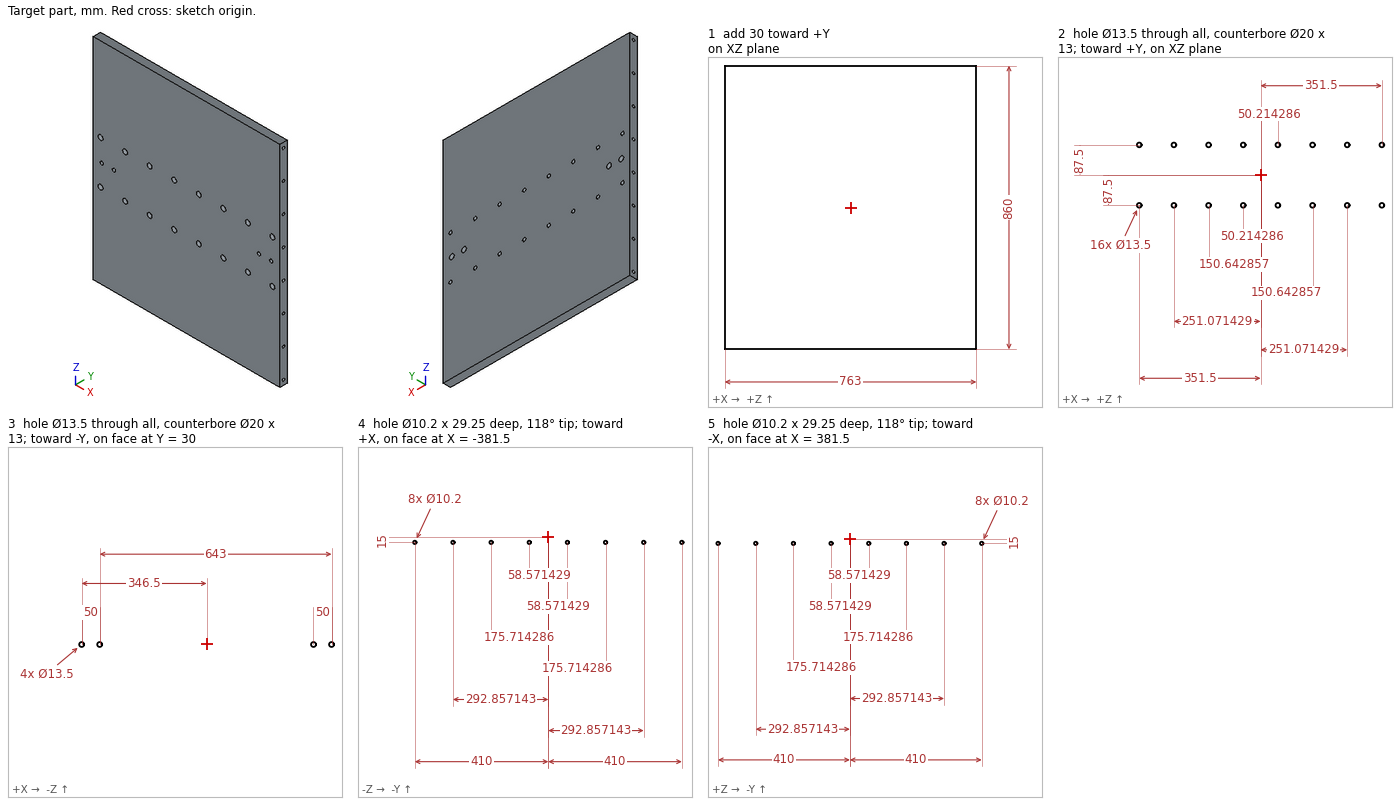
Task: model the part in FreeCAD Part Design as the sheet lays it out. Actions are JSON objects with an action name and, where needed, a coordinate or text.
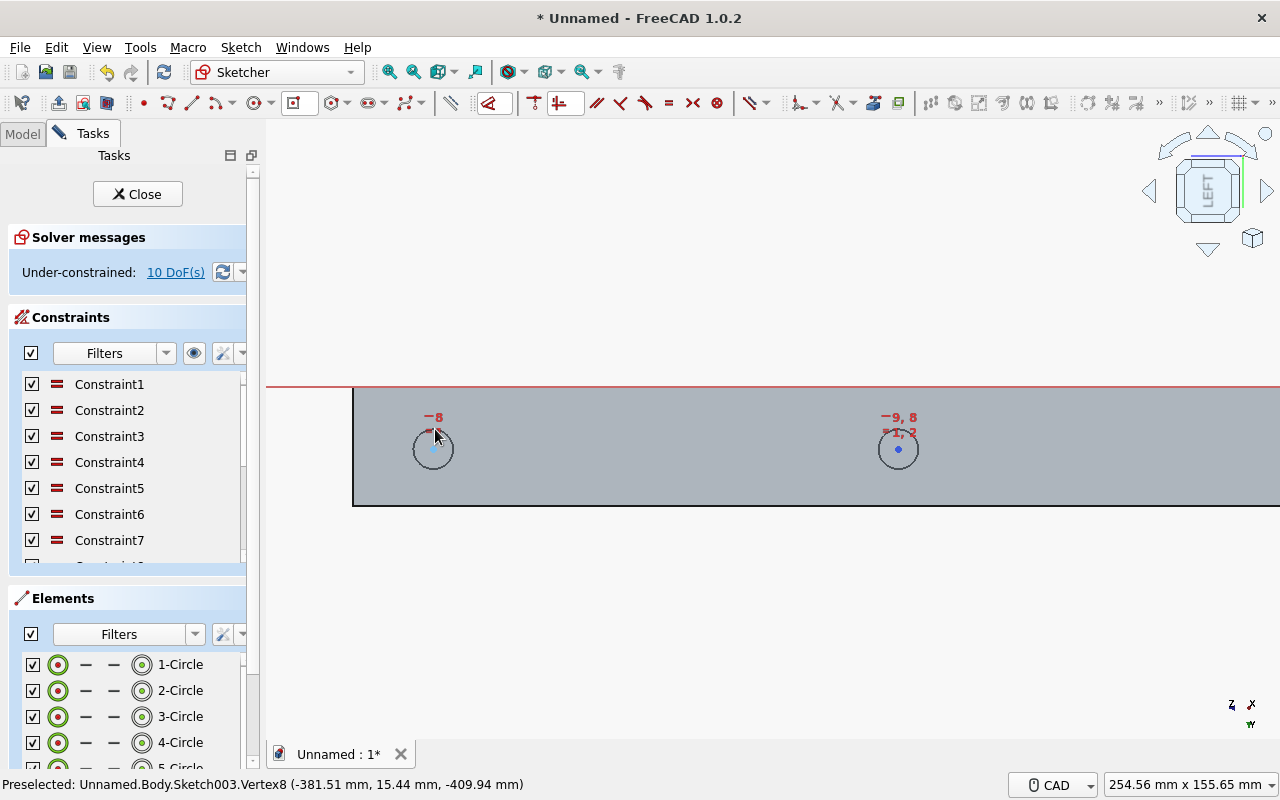
{"action": "left_click", "coordinate": [433, 469]}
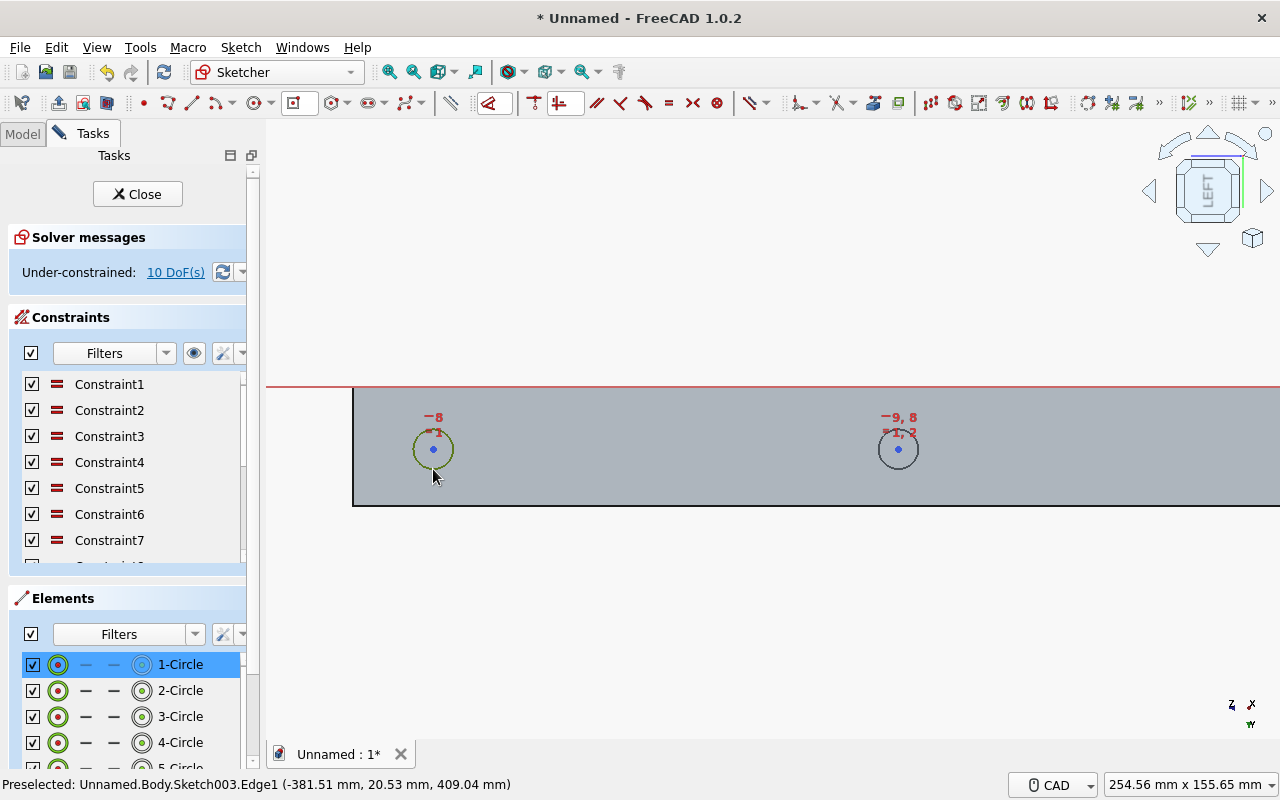
{"action": "key", "text": "k o"}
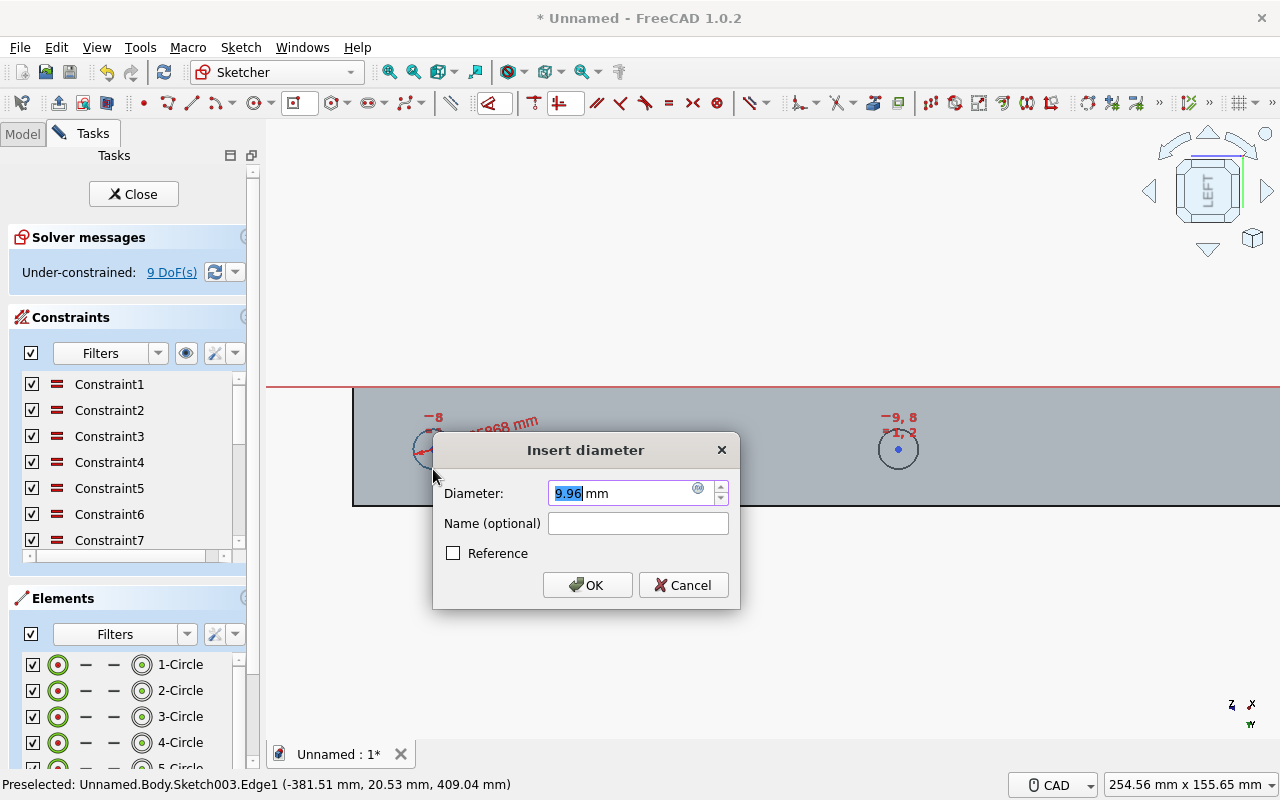
{"action": "type", "text": "10.2"}
{"action": "key", "text": "Return"}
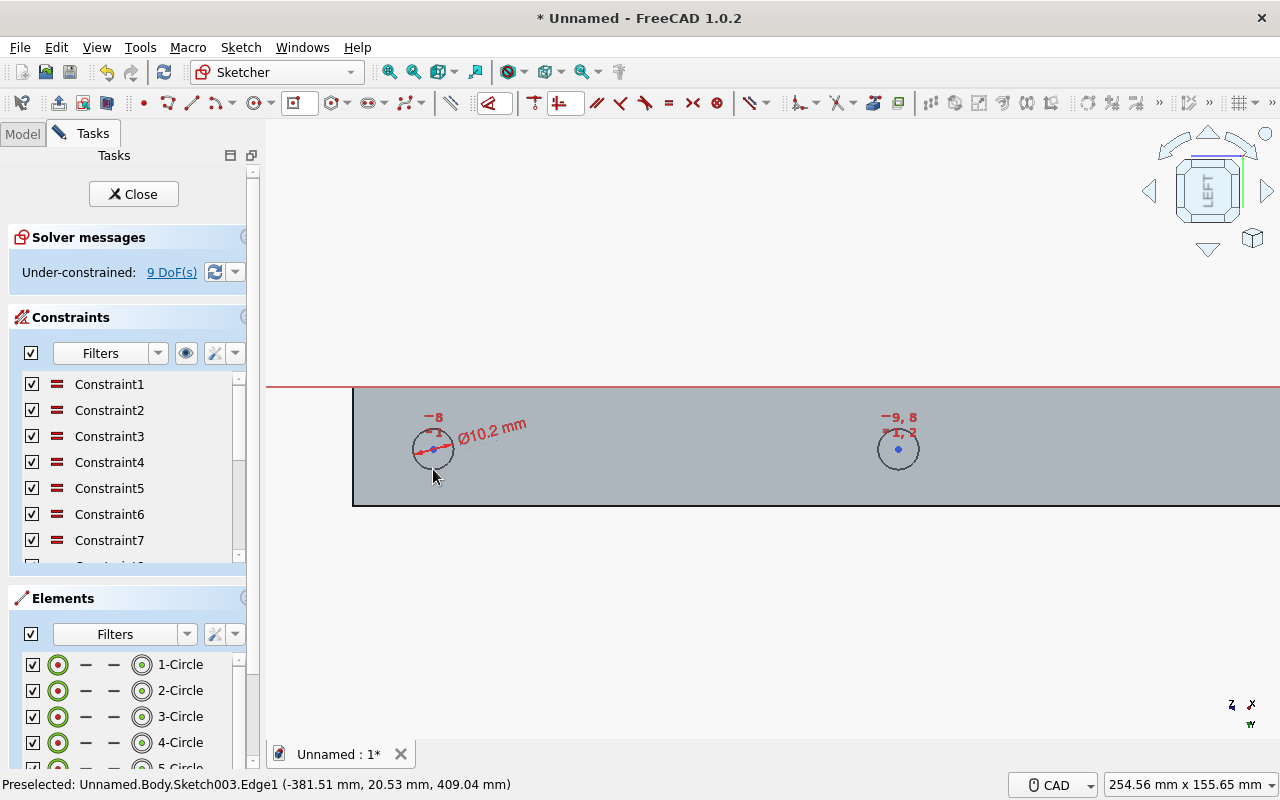
{"action": "left_click", "coordinate": [433, 449]}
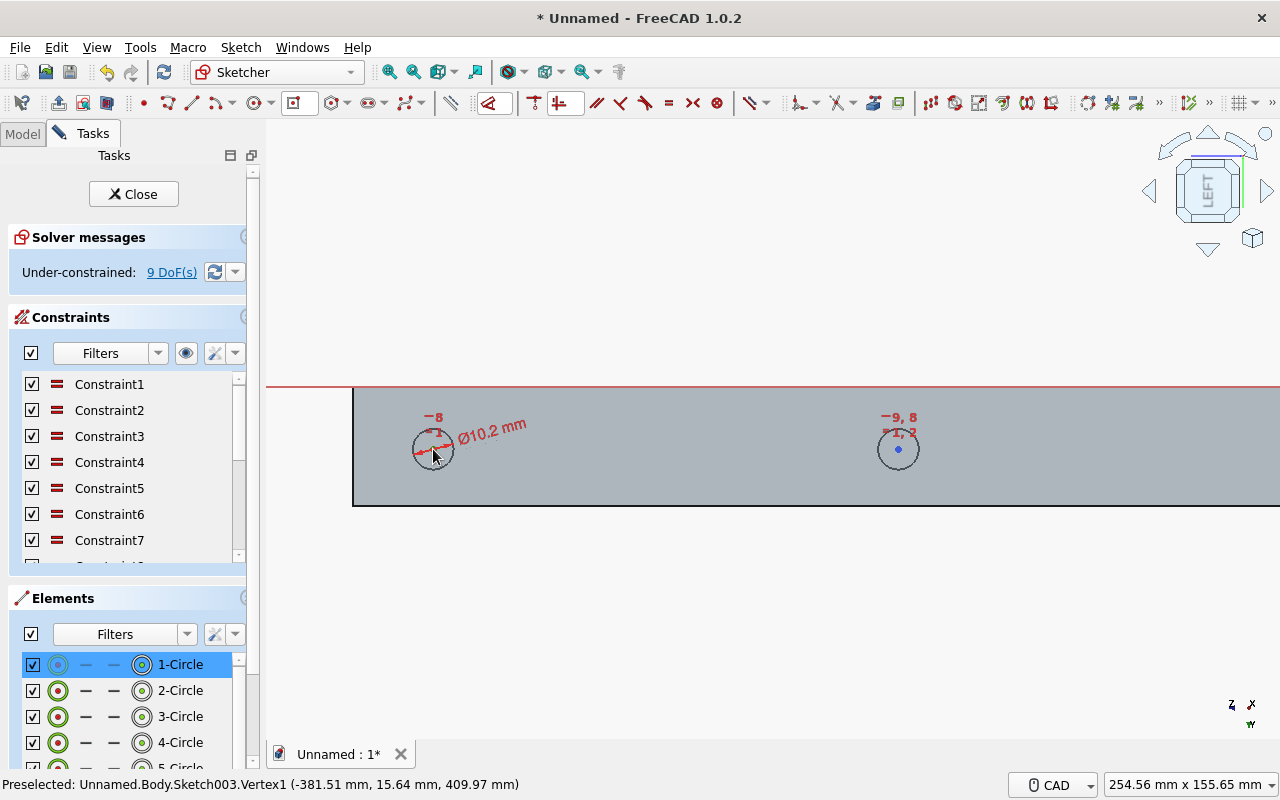
{"action": "key", "text": "i"}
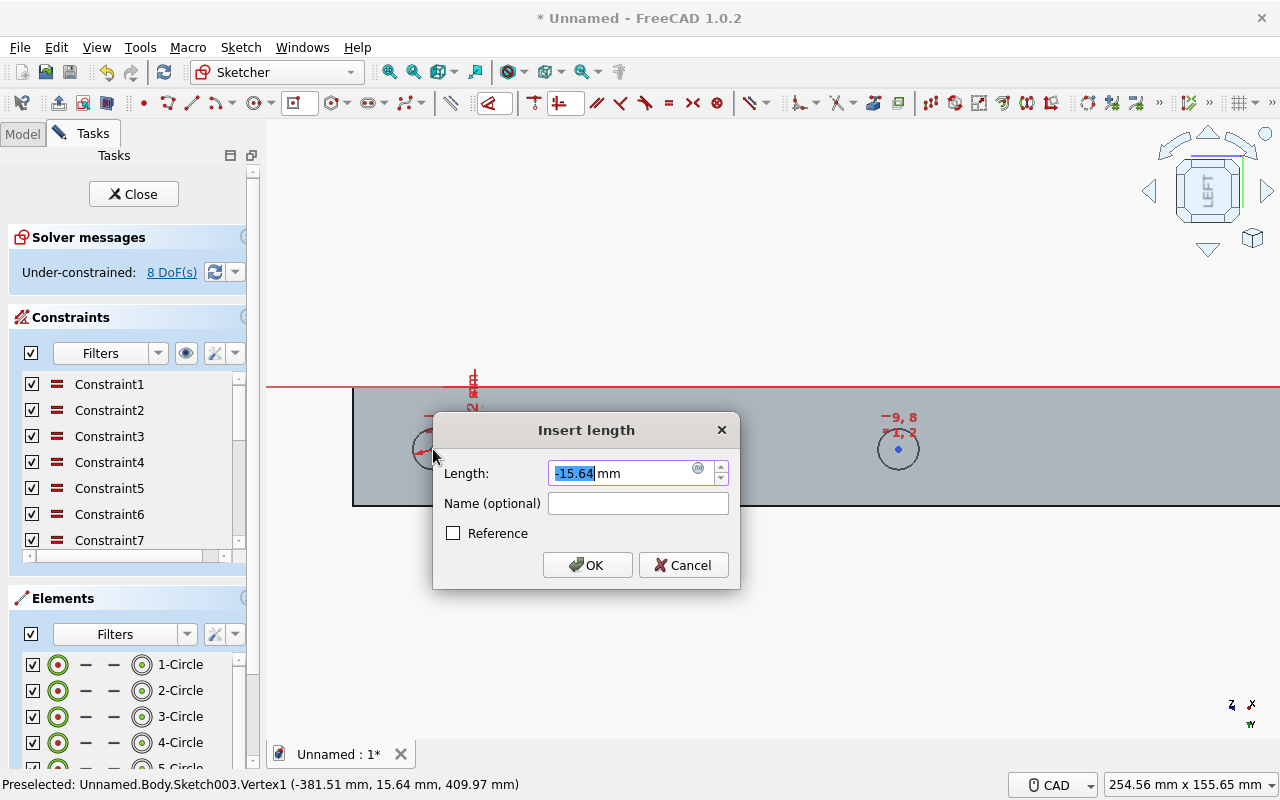
{"action": "type", "text": "-15"}
{"action": "key", "text": "Return"}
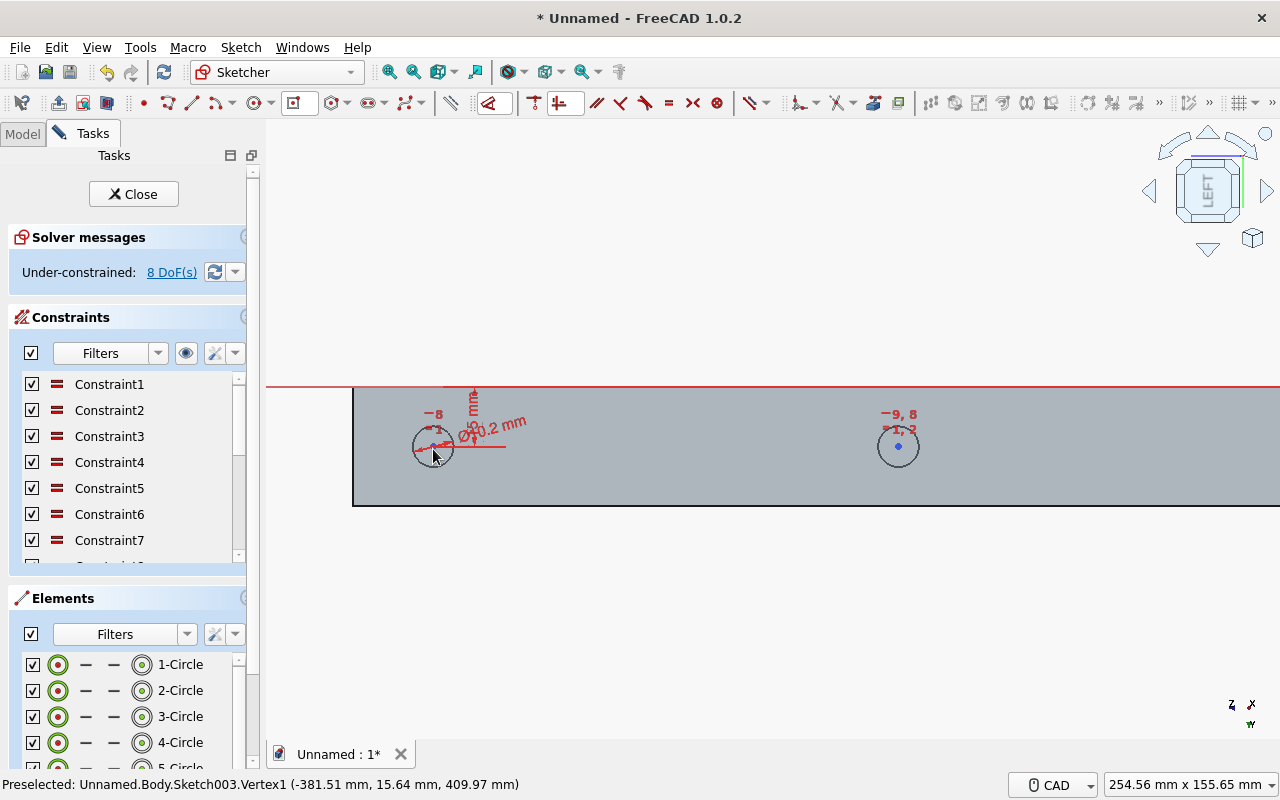
{"action": "scroll", "coordinate": [435, 429], "scroll_direction": "down", "scroll_amount": 9}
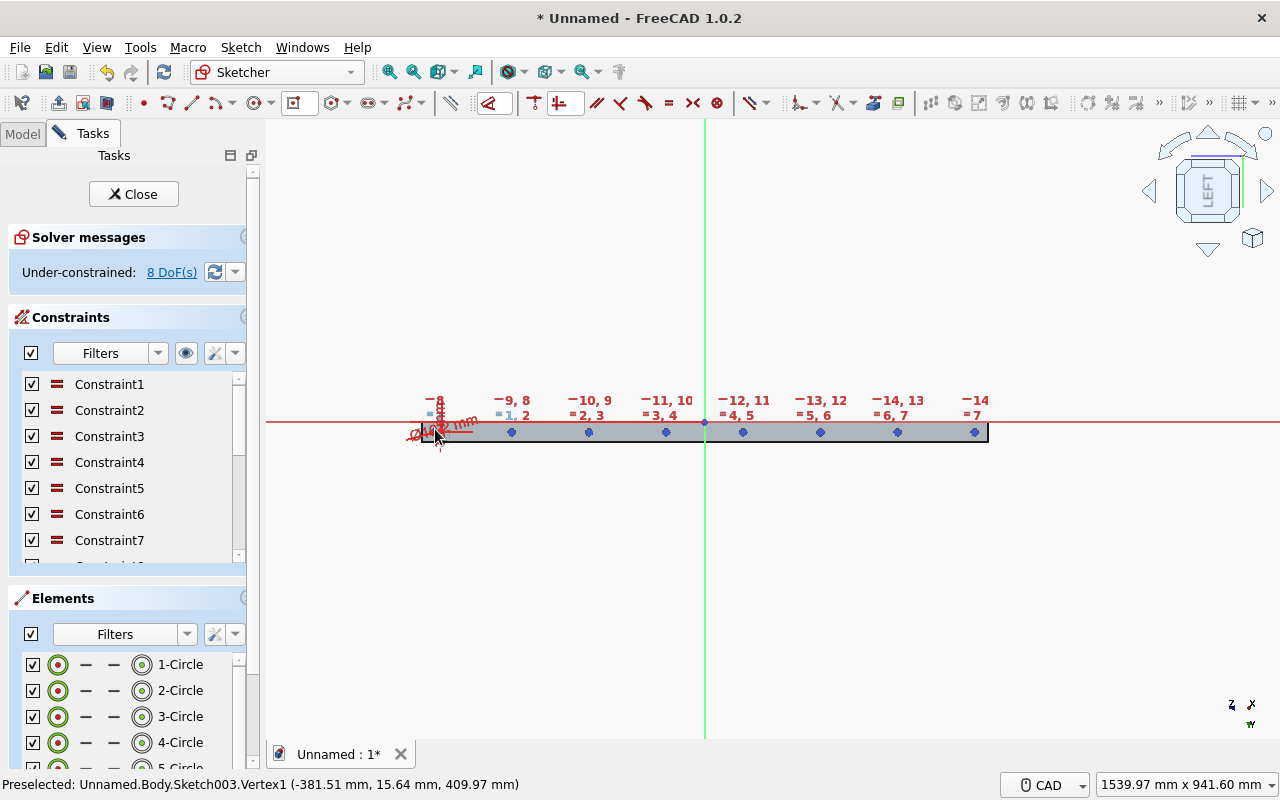
{"action": "left_click", "coordinate": [435, 432]}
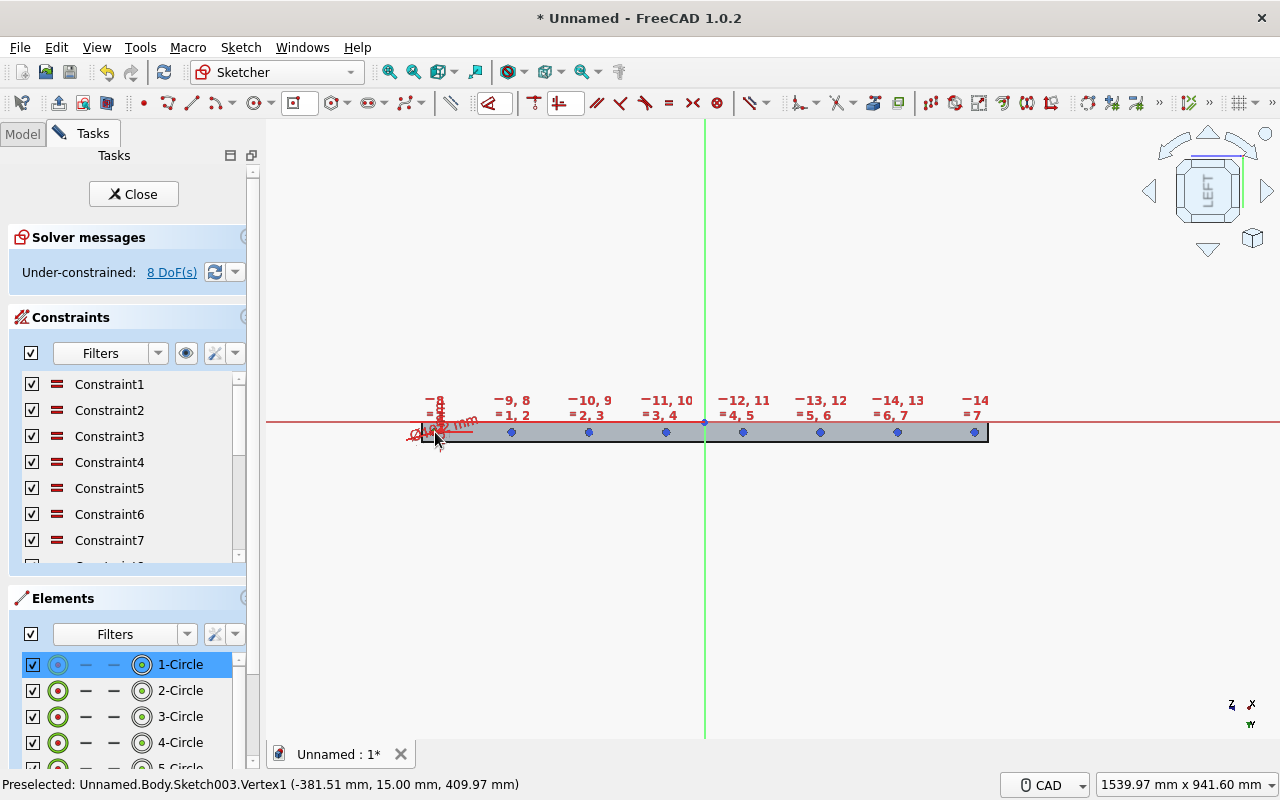
{"action": "key", "text": "l"}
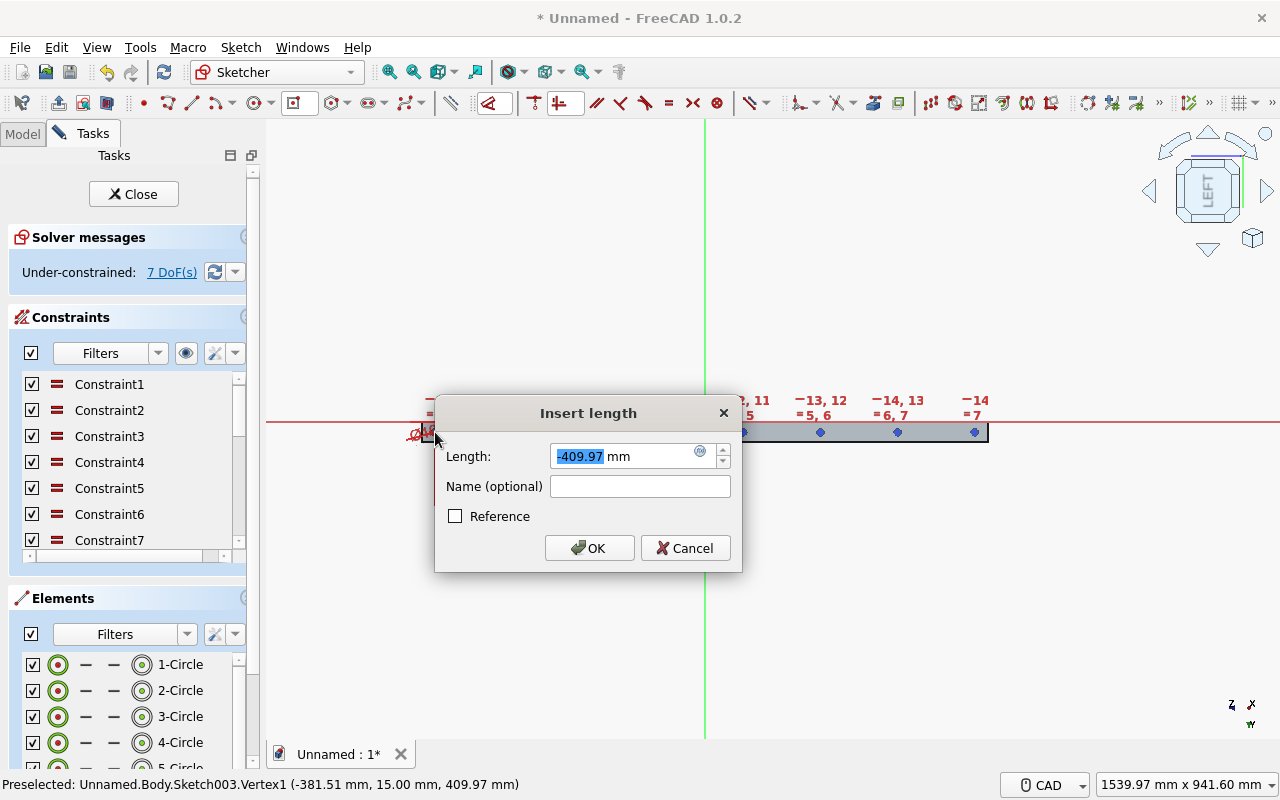
{"action": "type", "text": "-410"}
{"action": "key", "text": "Return"}